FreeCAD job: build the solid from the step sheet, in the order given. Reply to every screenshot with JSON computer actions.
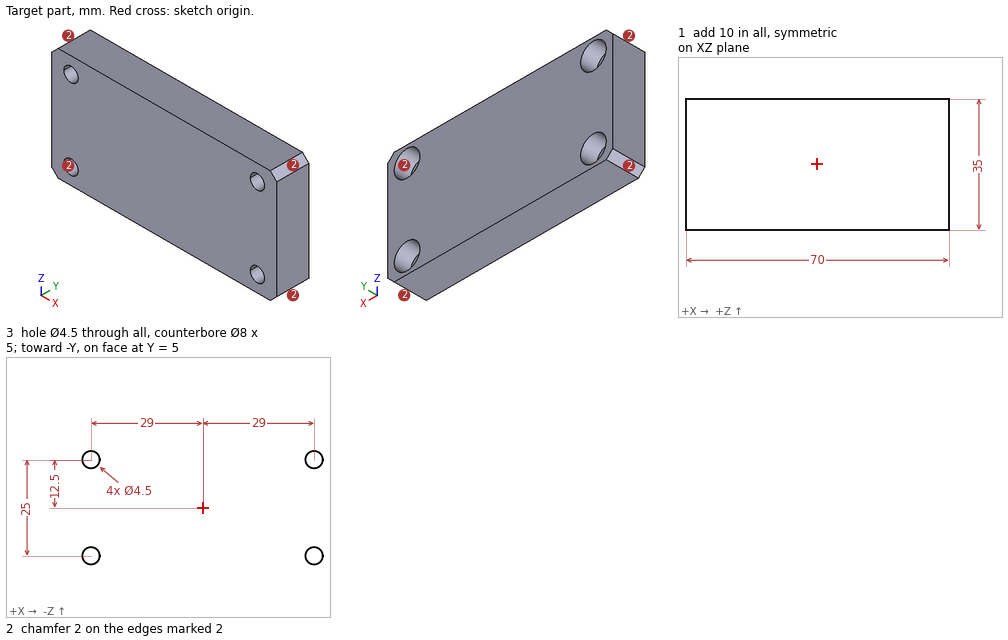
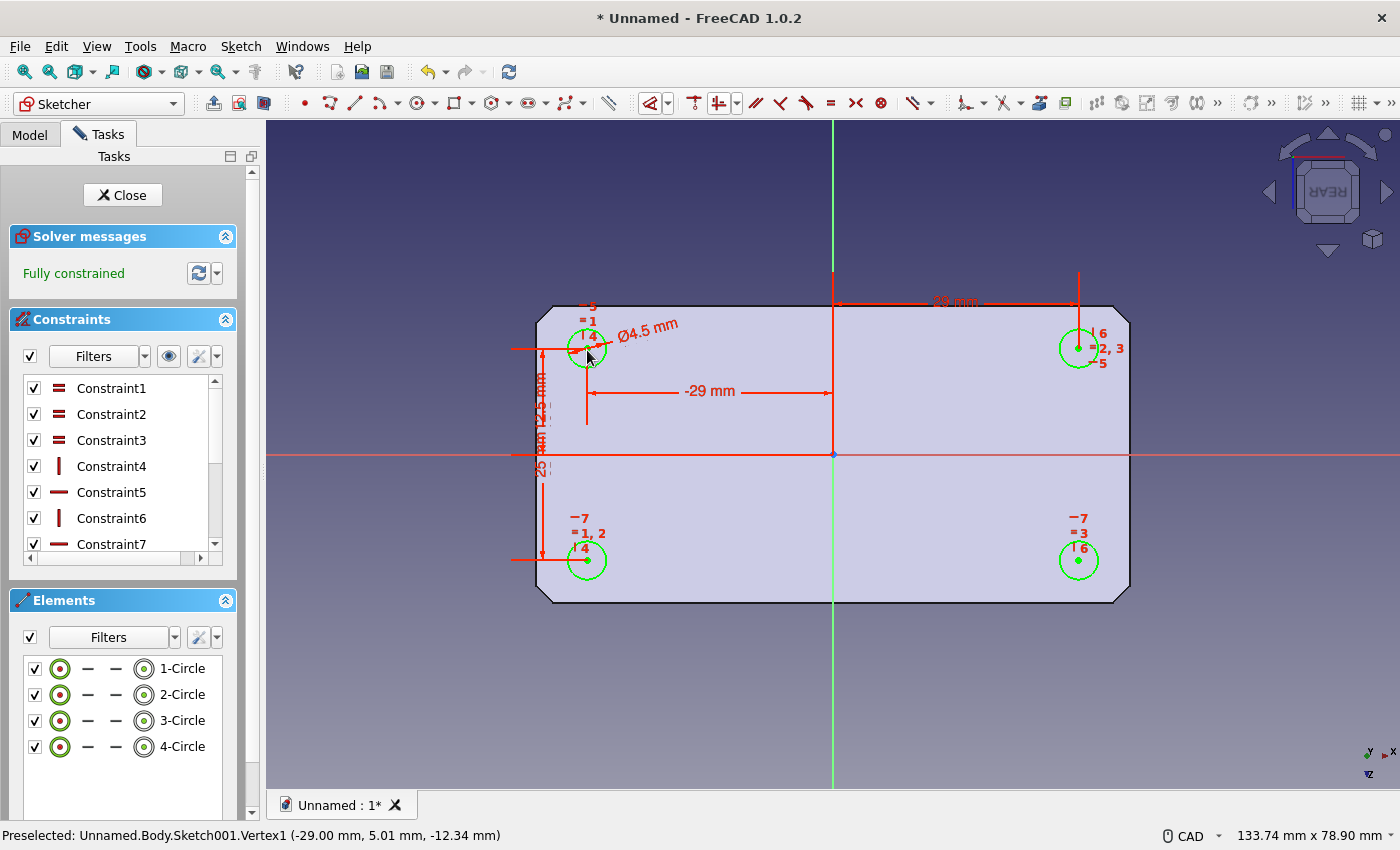
{"action": "left_click", "coordinate": [123, 195]}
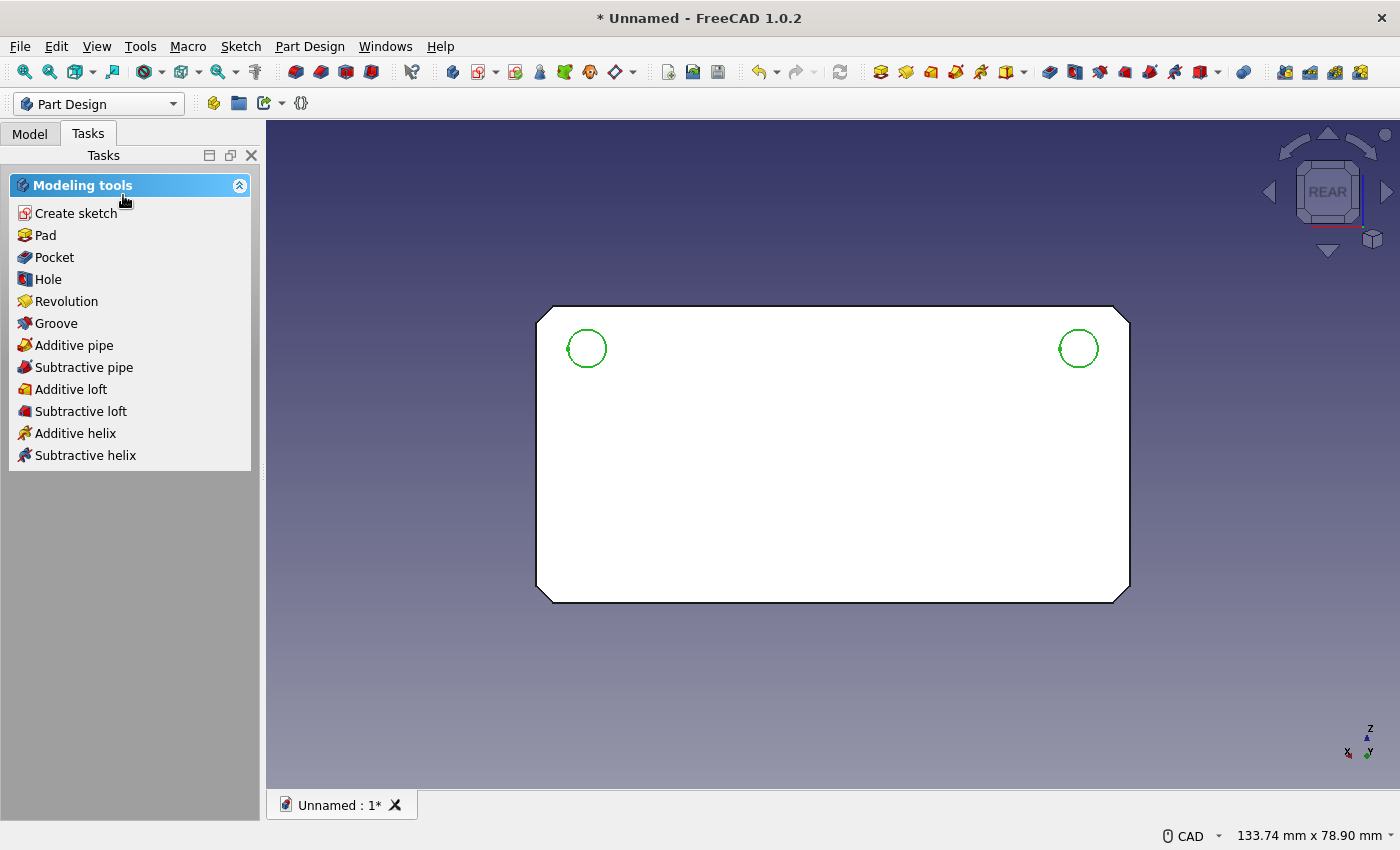
{"action": "left_click", "coordinate": [1075, 72]}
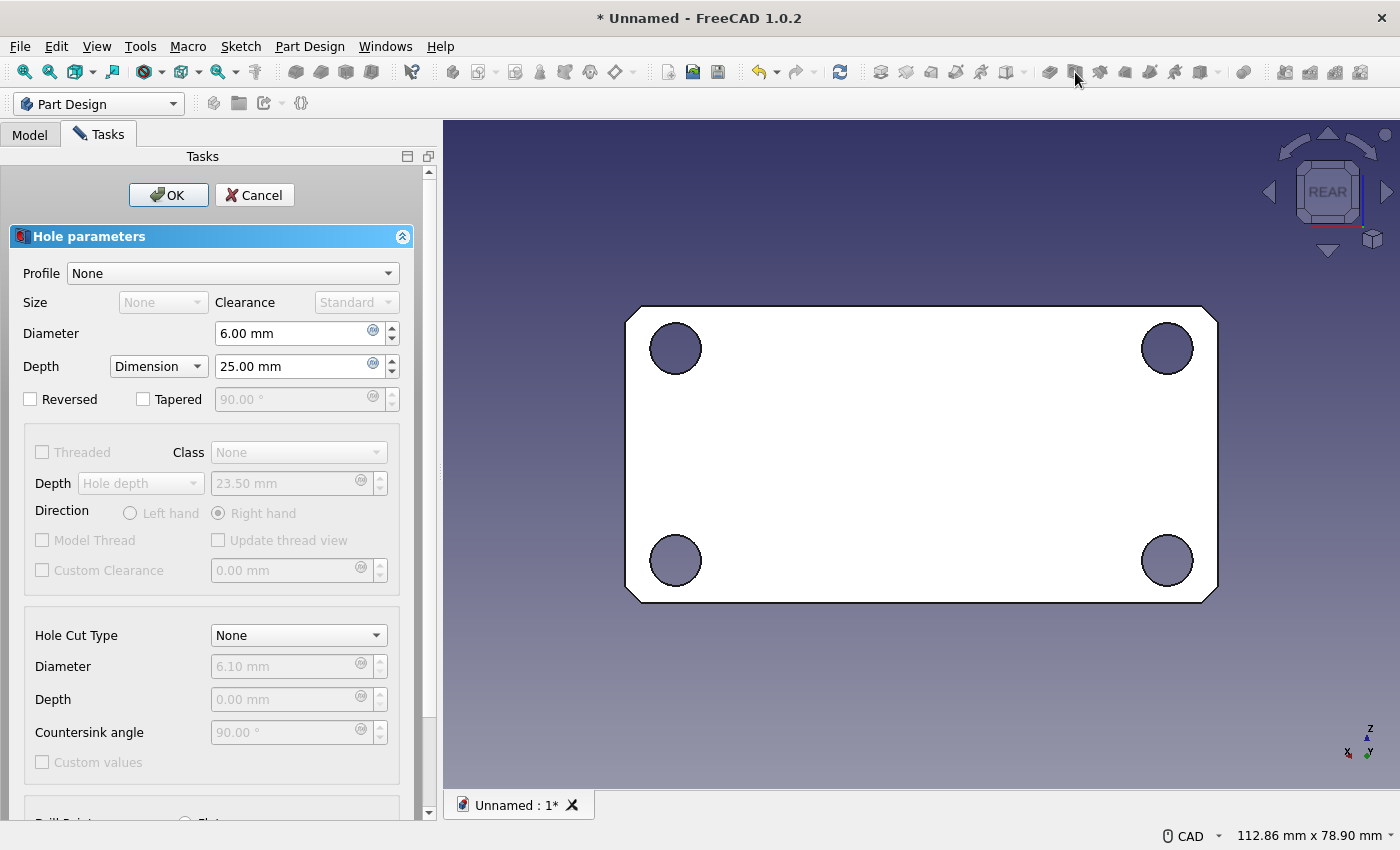
{"action": "triple_click", "coordinate": [300, 334]}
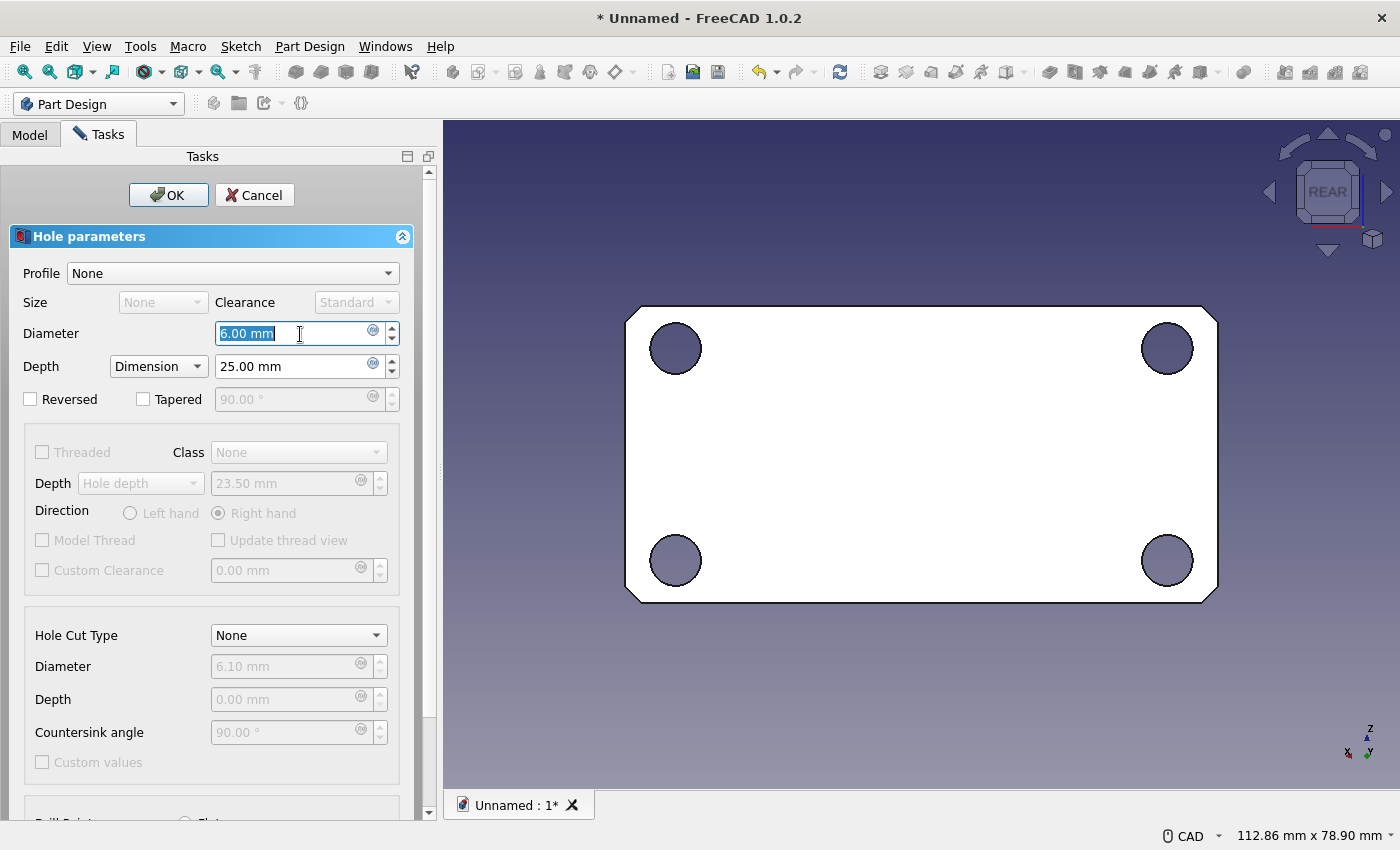
{"action": "type", "text": "4.5"}
{"action": "key", "text": "Tab"}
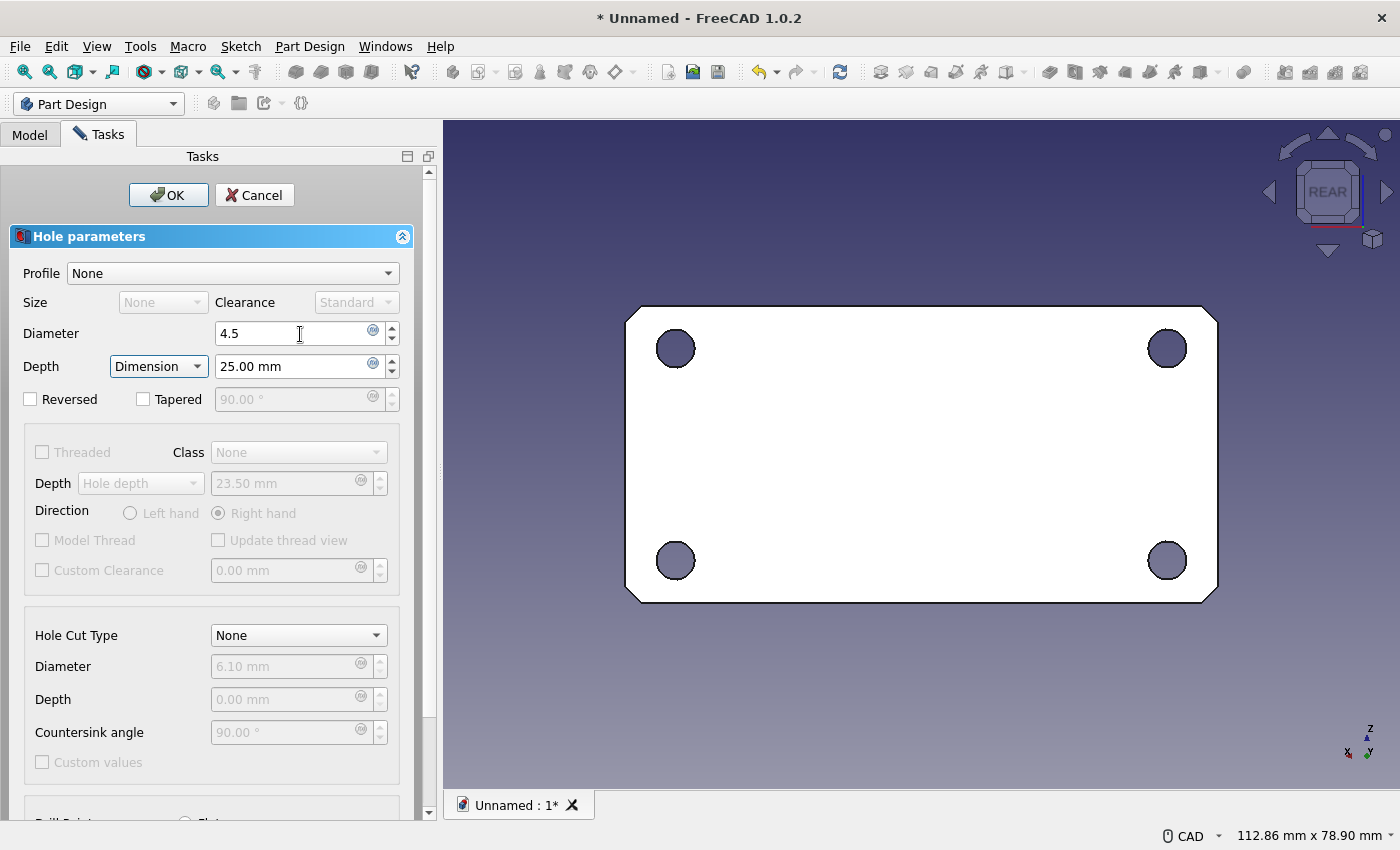
{"action": "left_click", "coordinate": [160, 366]}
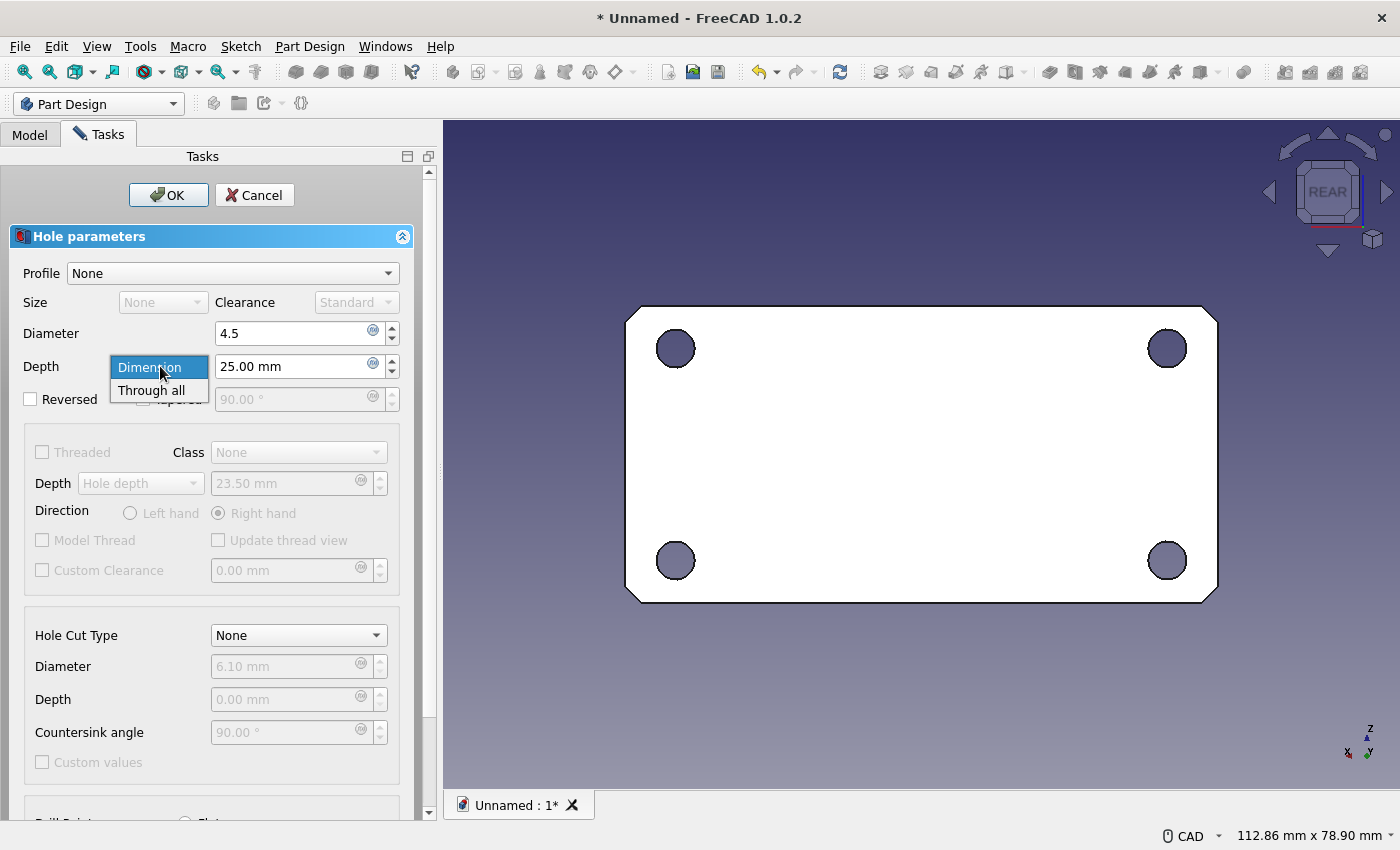
{"action": "left_click", "coordinate": [158, 390]}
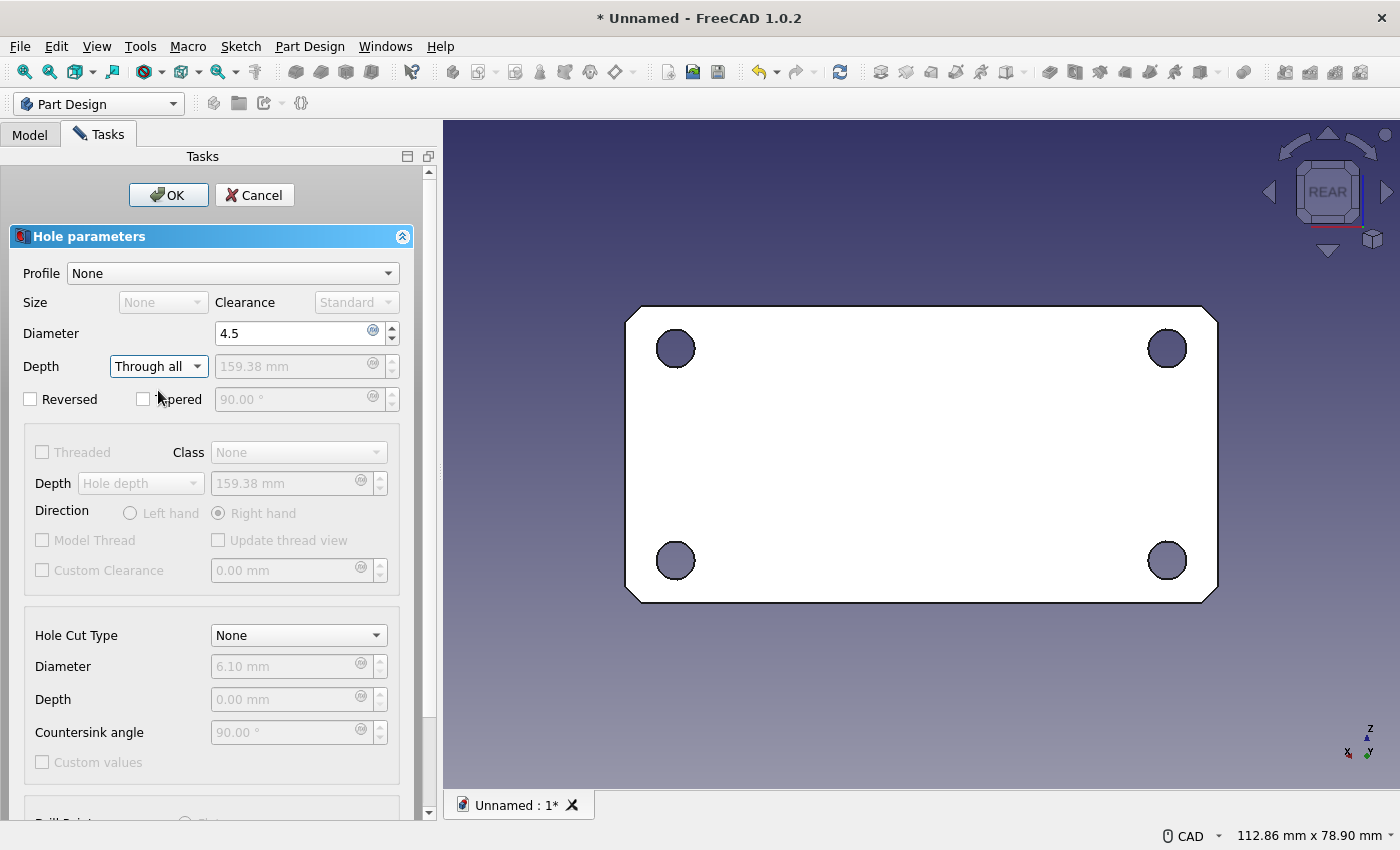
{"action": "left_click", "coordinate": [300, 636]}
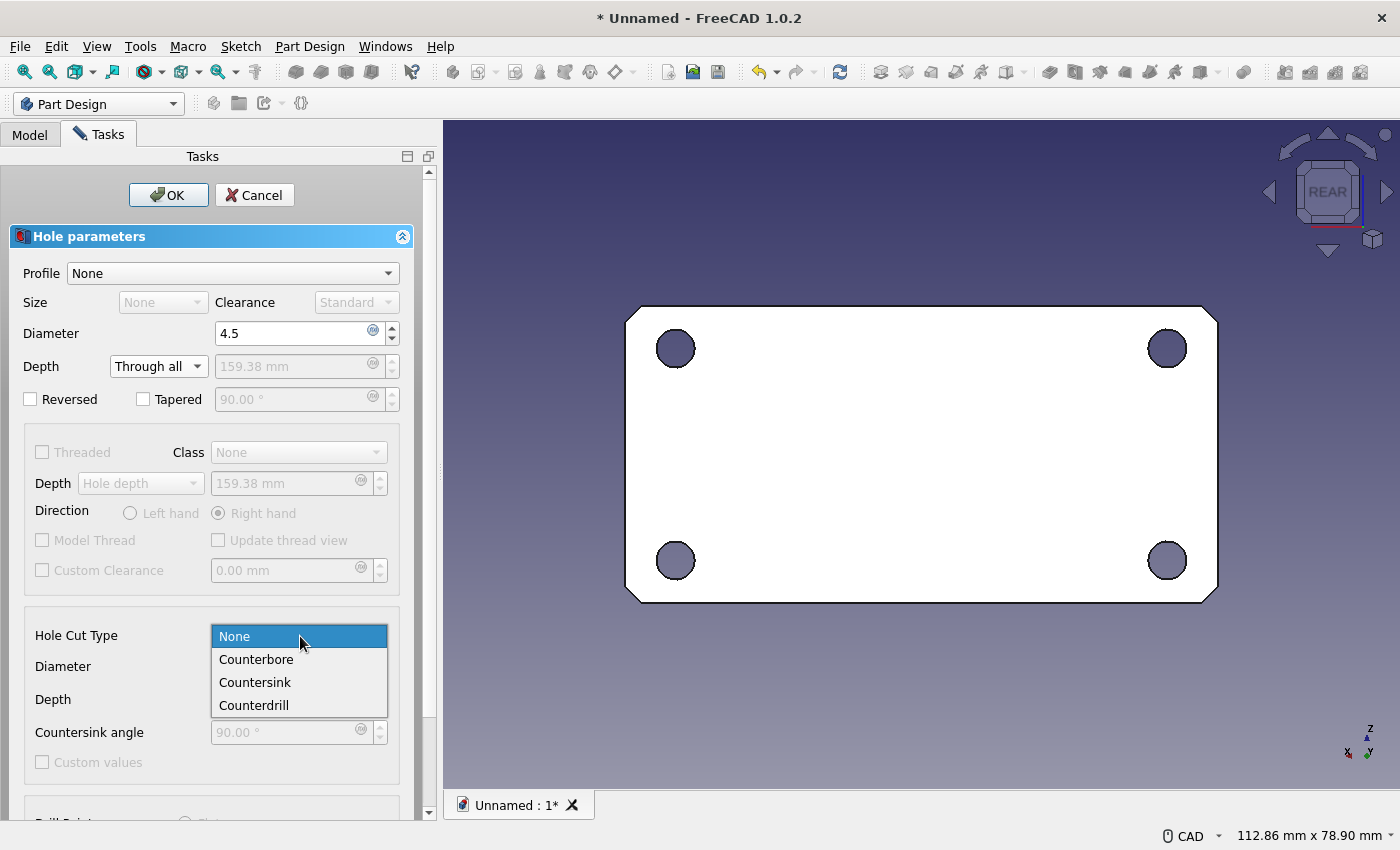
{"action": "left_click", "coordinate": [298, 660]}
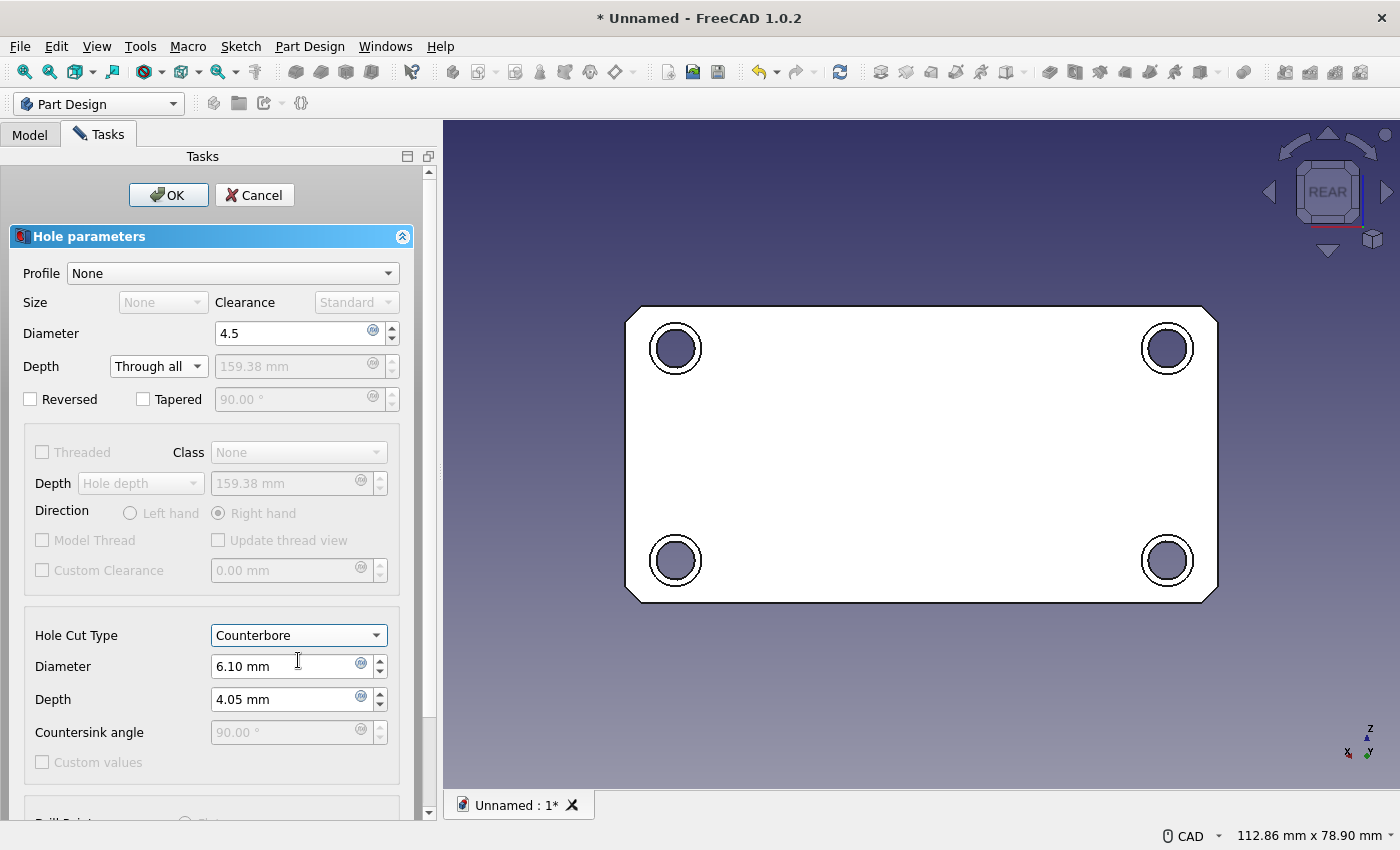
{"action": "triple_click", "coordinate": [292, 666]}